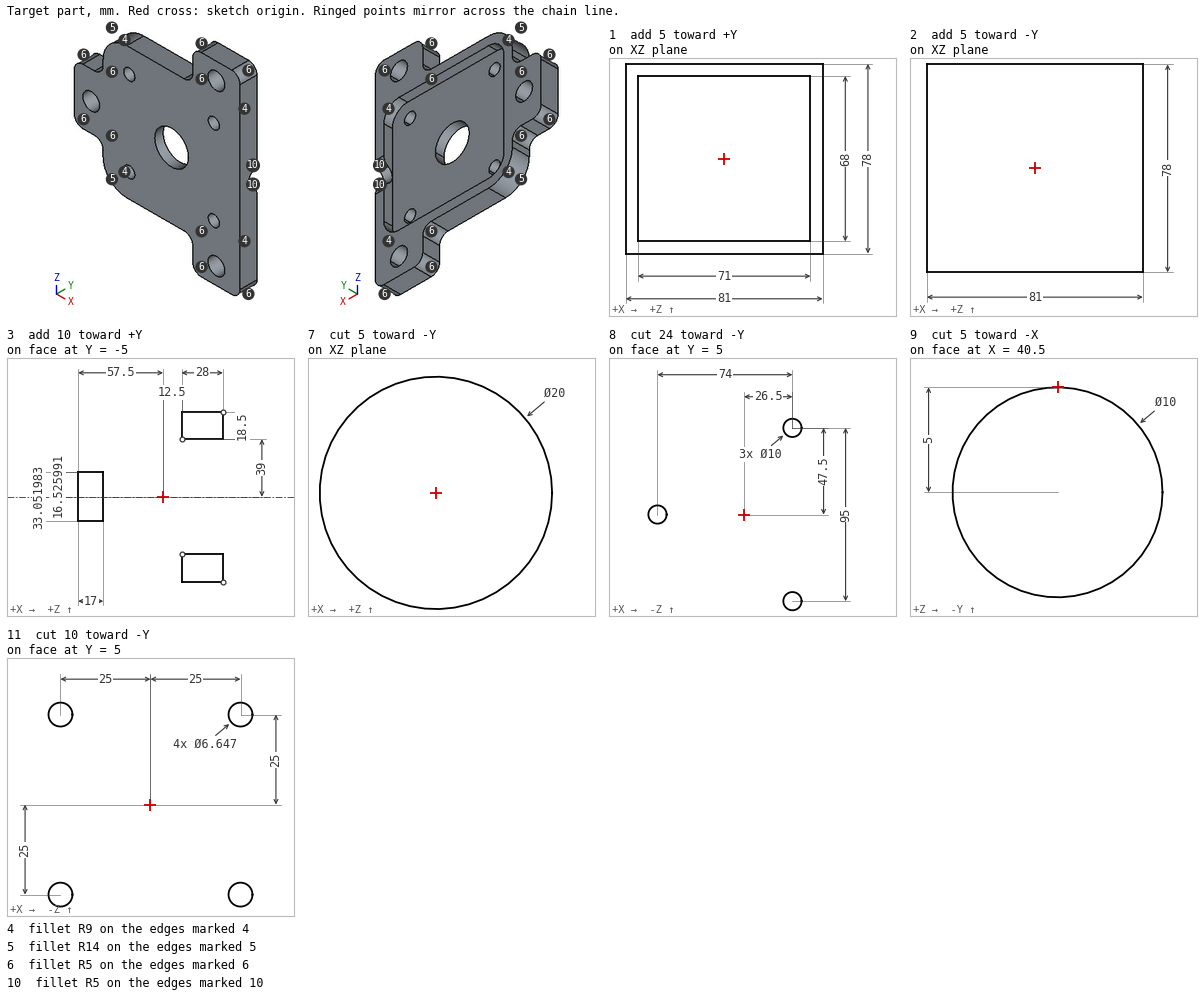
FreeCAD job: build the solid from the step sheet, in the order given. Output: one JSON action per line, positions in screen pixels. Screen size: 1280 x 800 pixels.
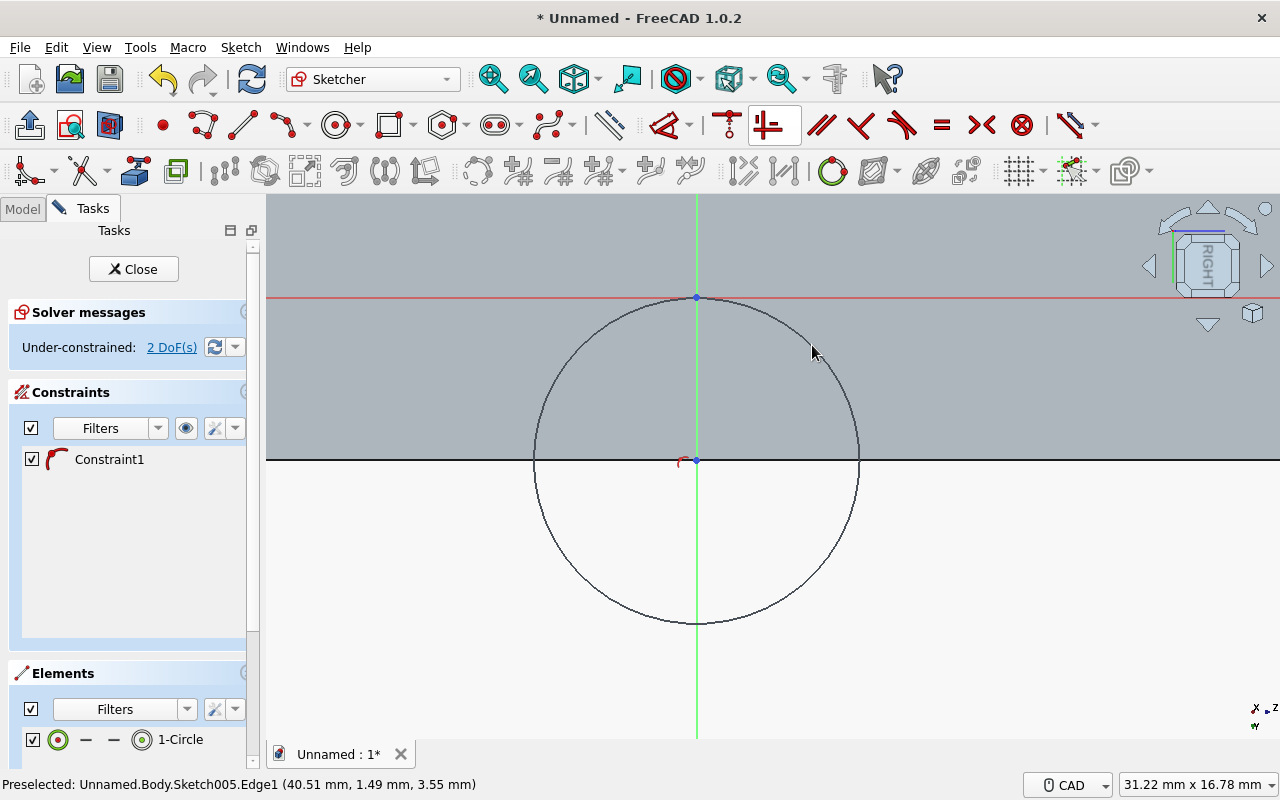
{"action": "left_click", "coordinate": [664, 126]}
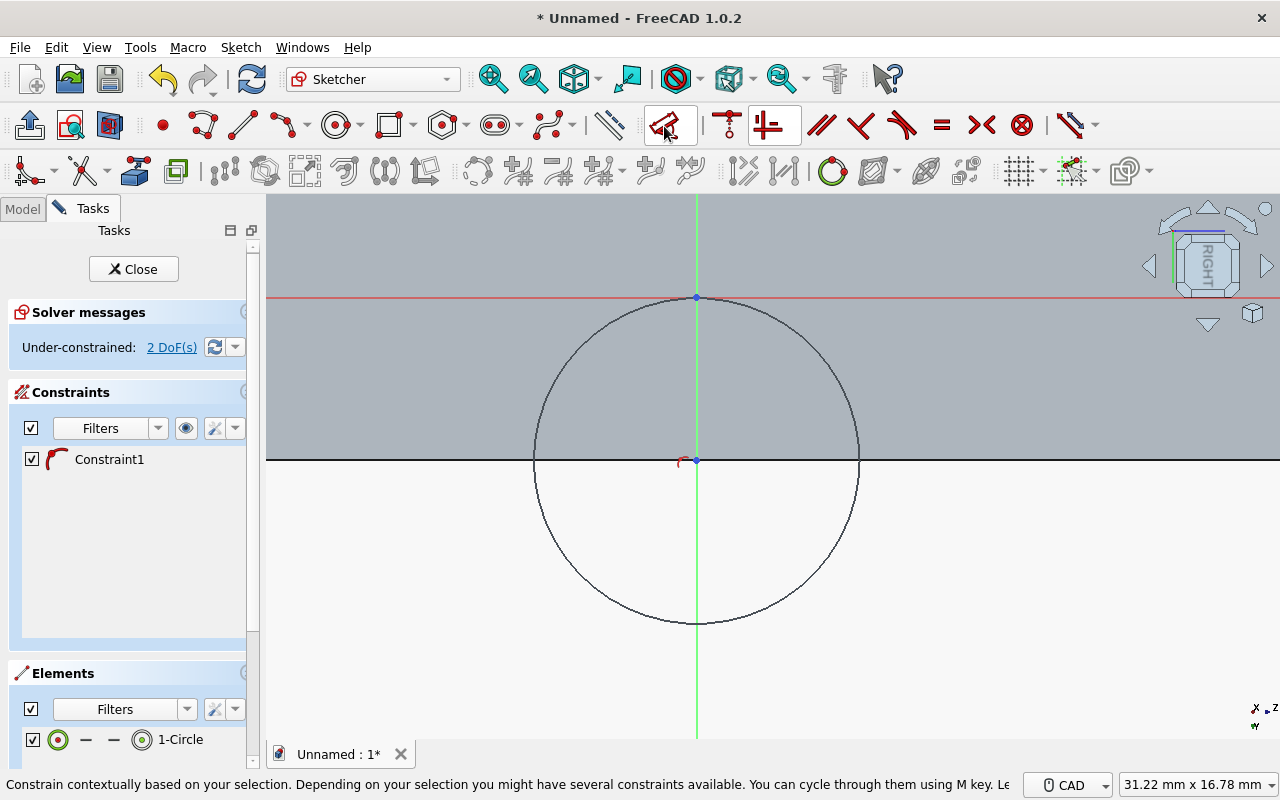
{"action": "left_click", "coordinate": [811, 345]}
{"action": "left_click", "coordinate": [833, 322]}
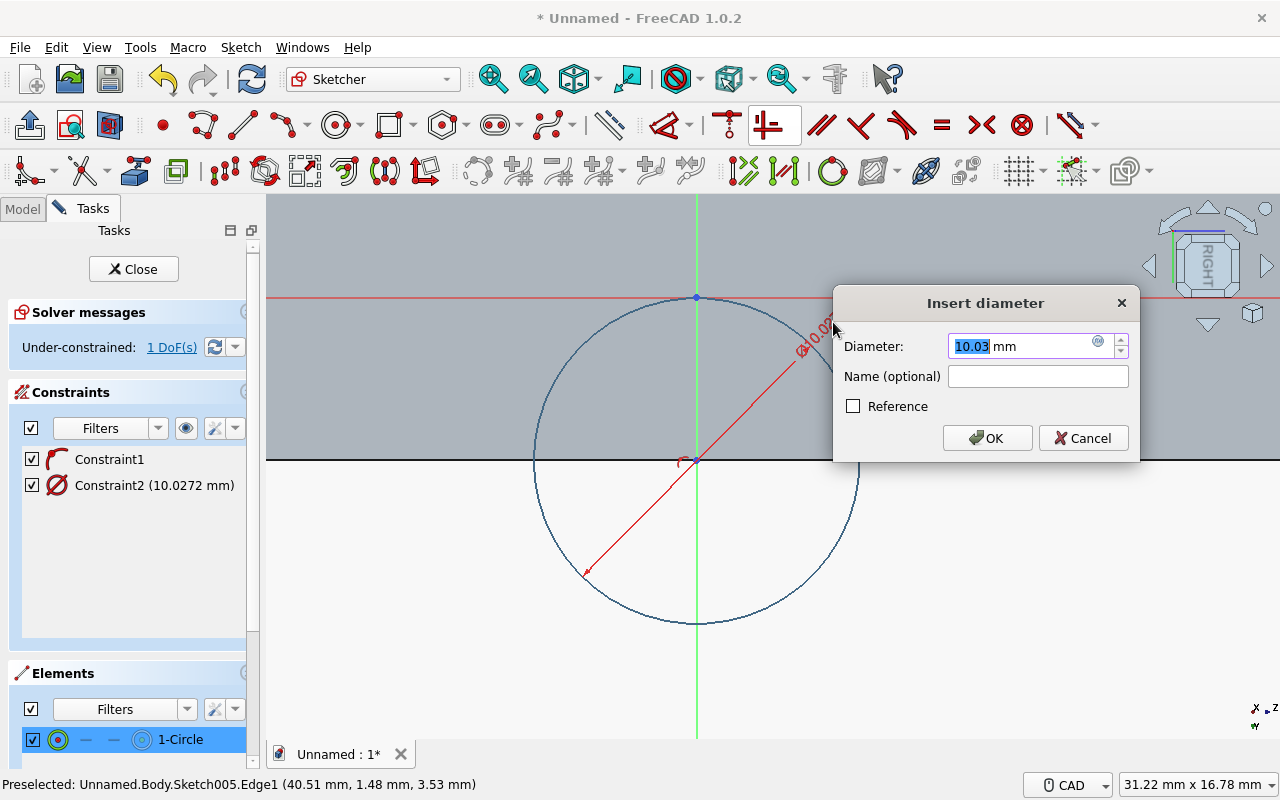
{"action": "type", "text": "10"}
{"action": "key", "text": "Return"}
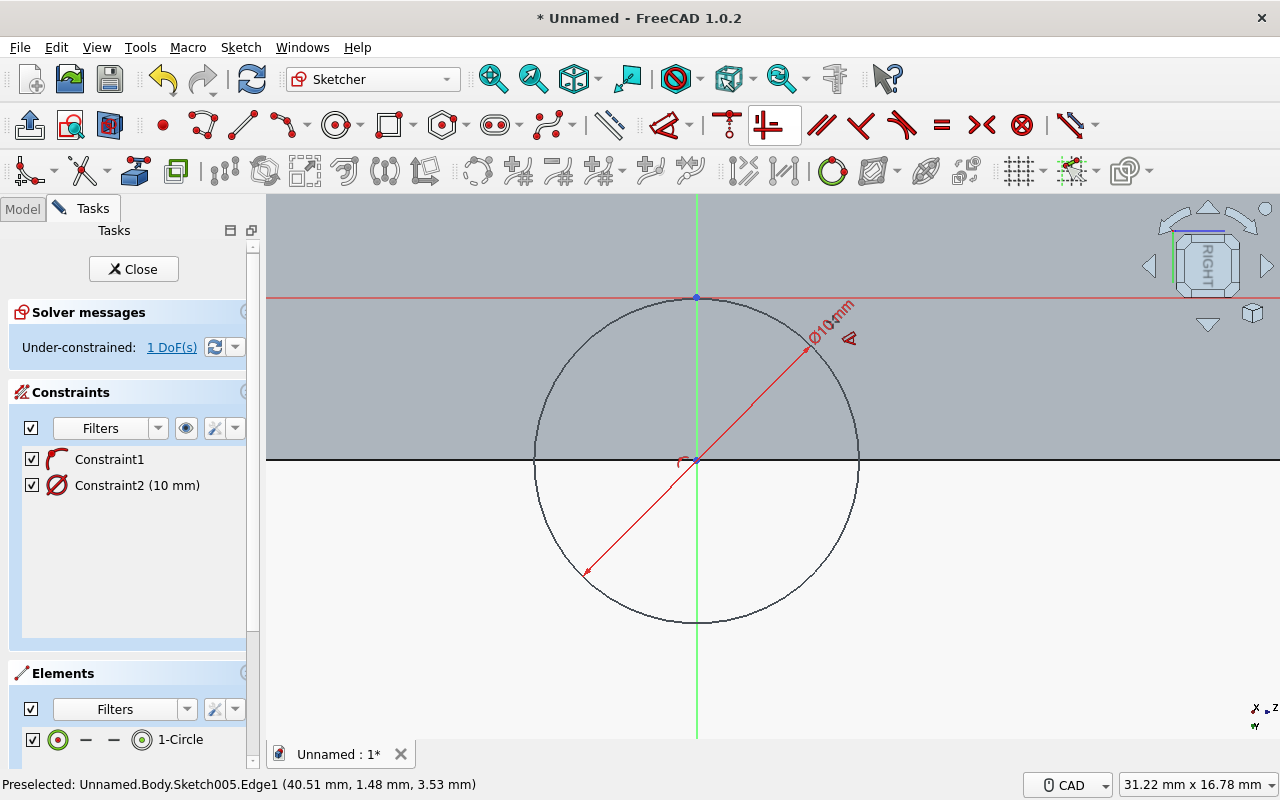
{"action": "left_click", "coordinate": [697, 461]}
{"action": "left_click", "coordinate": [731, 379]}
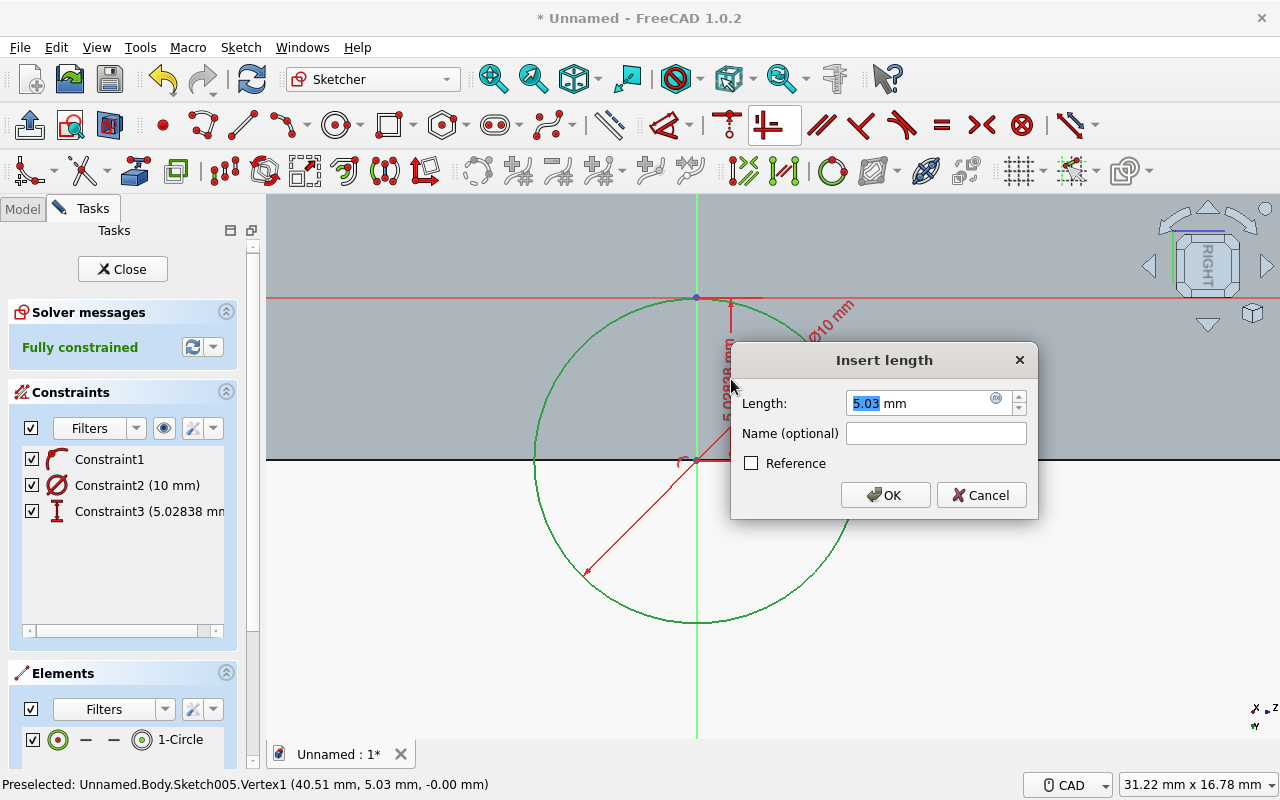
{"action": "type", "text": "5"}
{"action": "key", "text": "Return"}
{"action": "key", "text": "Escape"}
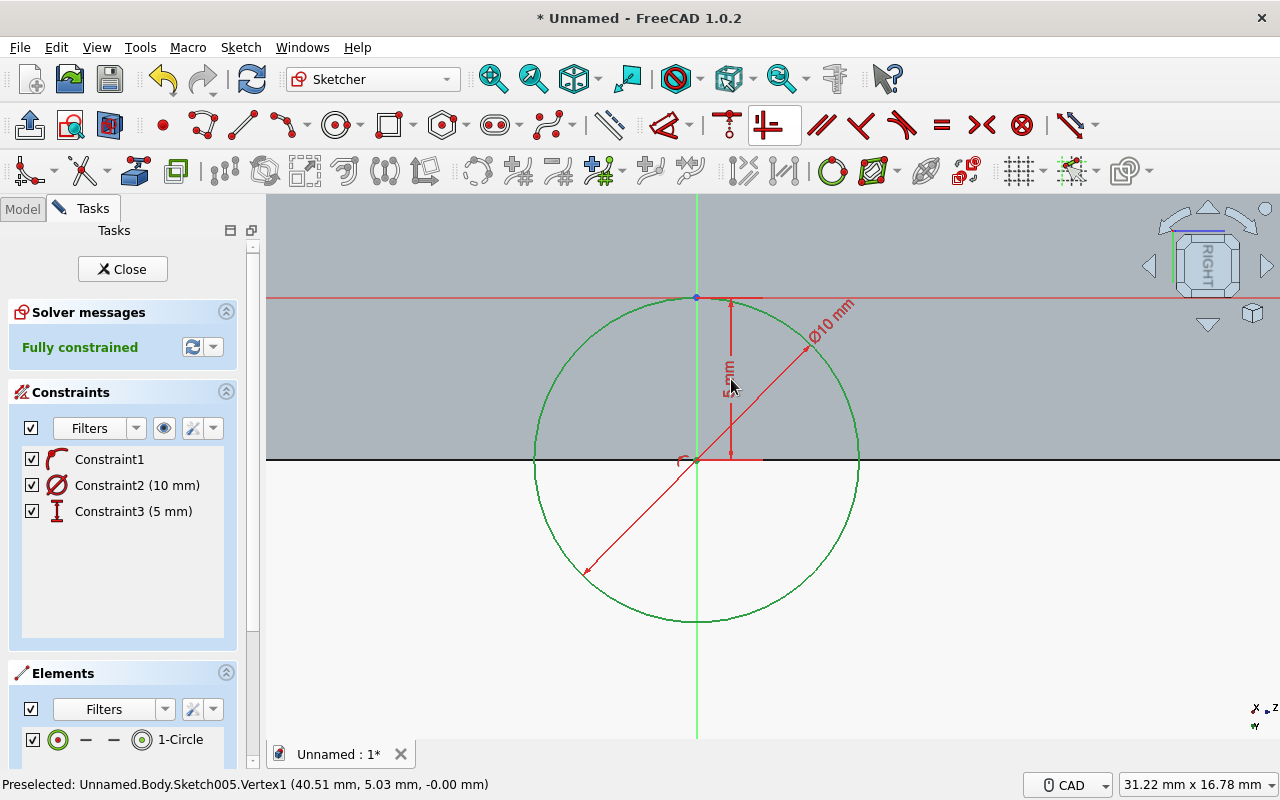
{"action": "left_click", "coordinate": [123, 269]}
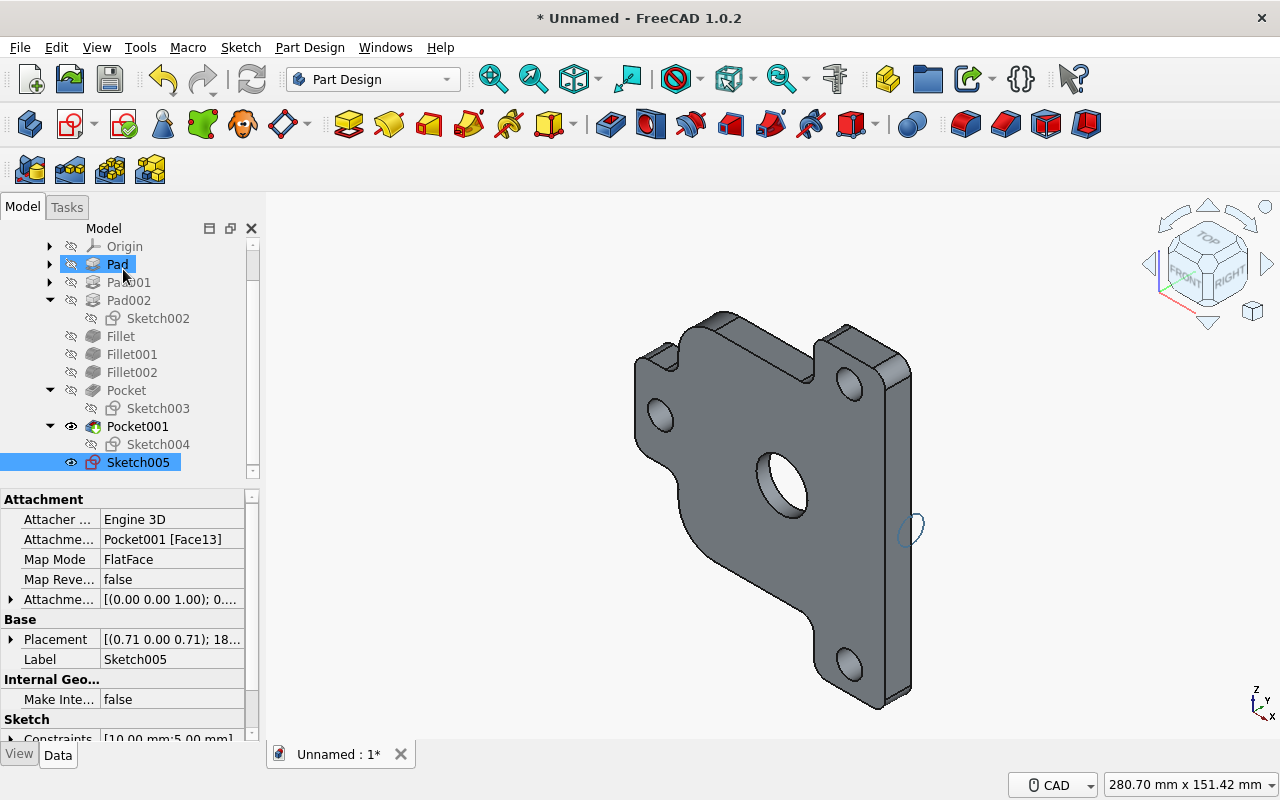
{"action": "left_click", "coordinate": [612, 124]}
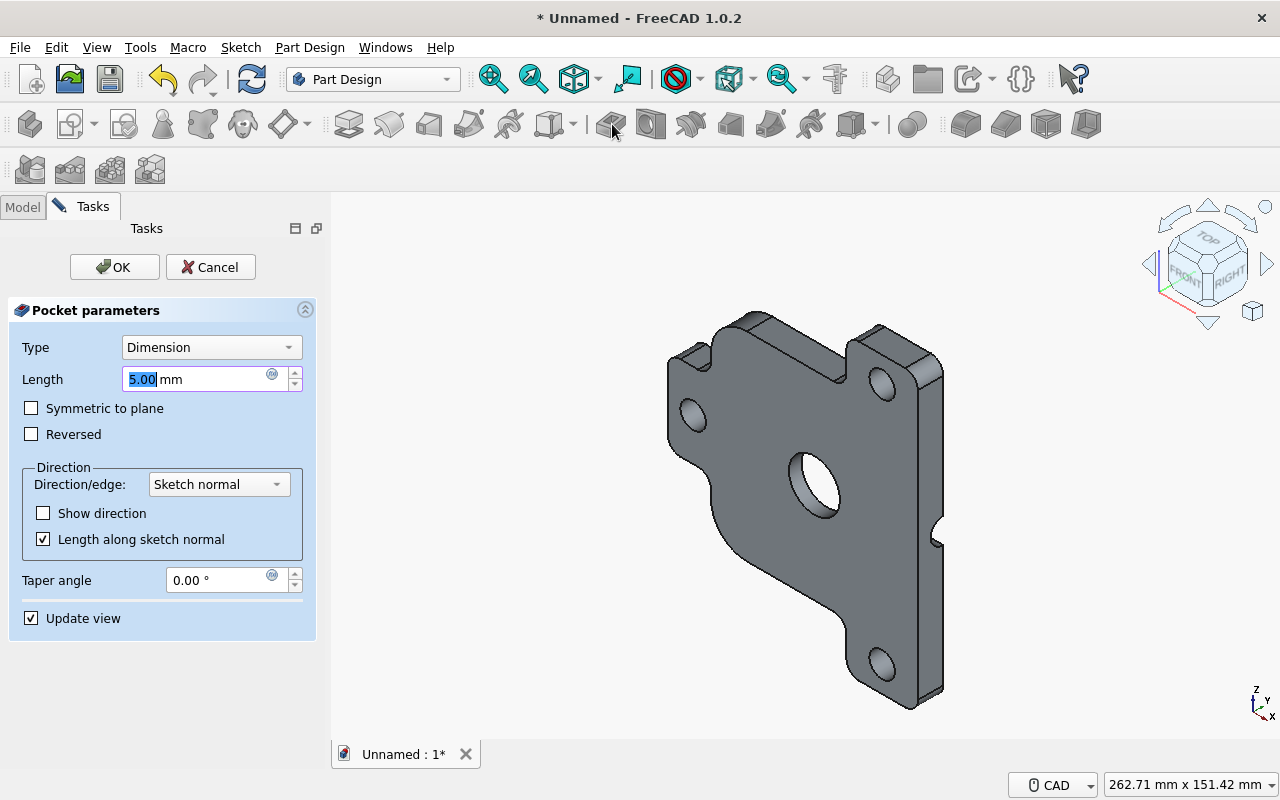
{"action": "type", "text": "5"}
{"action": "key", "text": "Tab"}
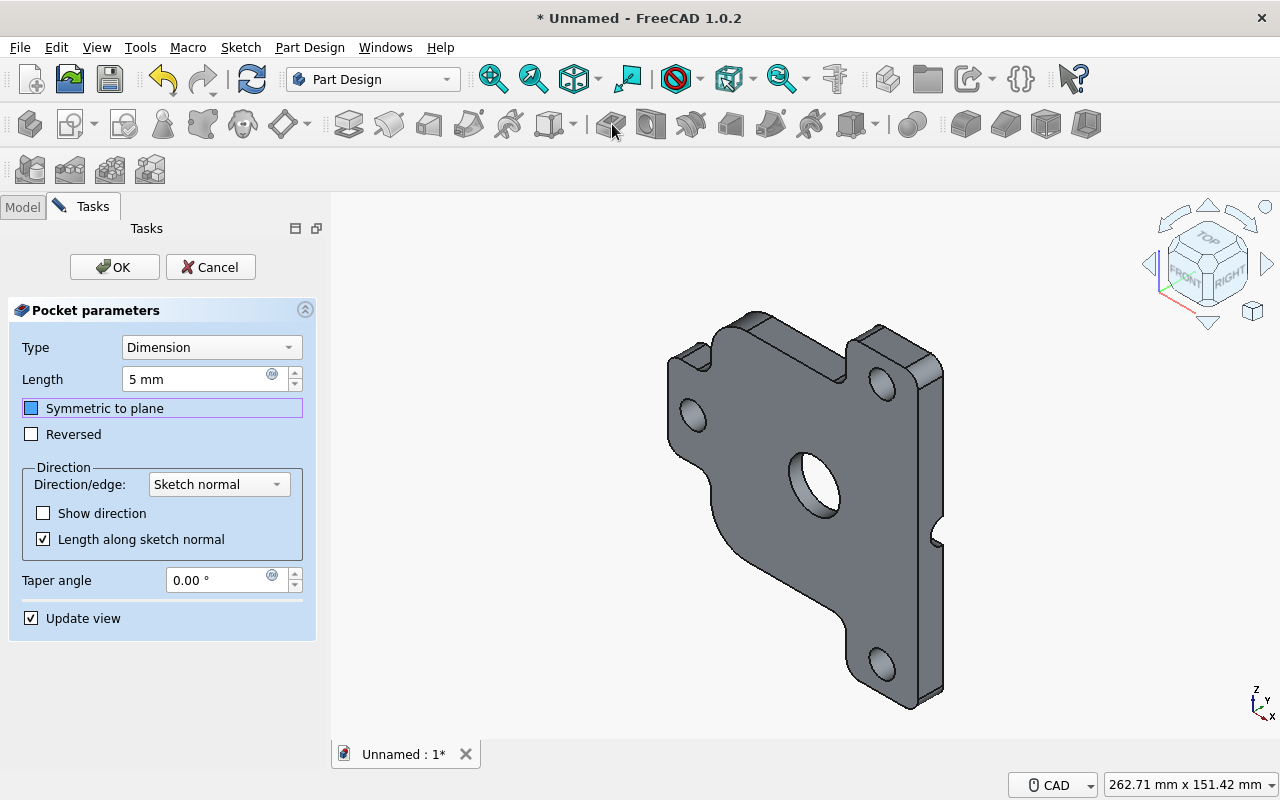
{"action": "left_click", "coordinate": [115, 267]}